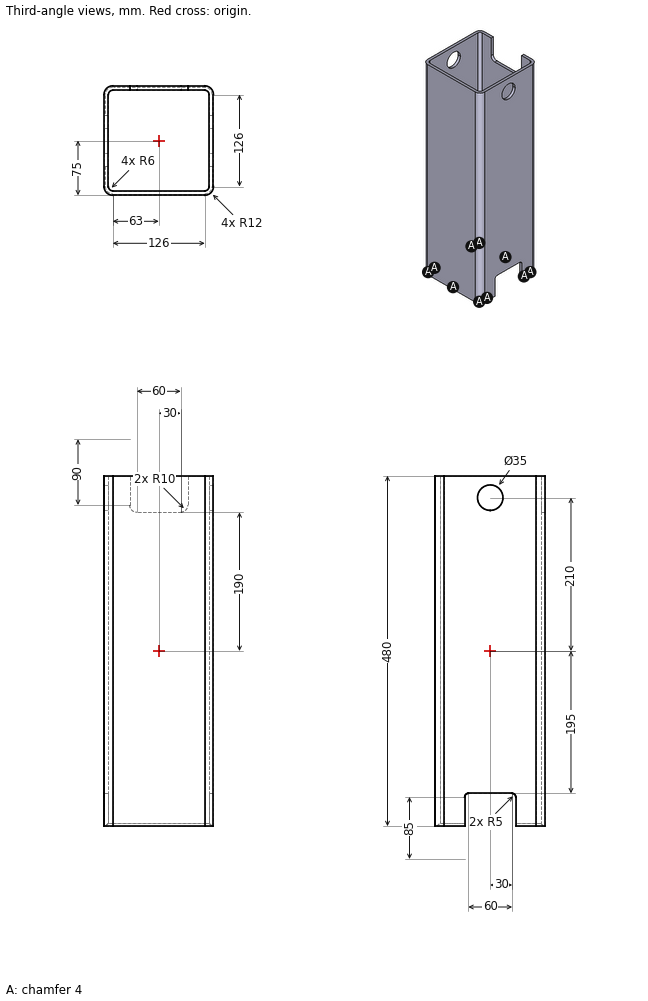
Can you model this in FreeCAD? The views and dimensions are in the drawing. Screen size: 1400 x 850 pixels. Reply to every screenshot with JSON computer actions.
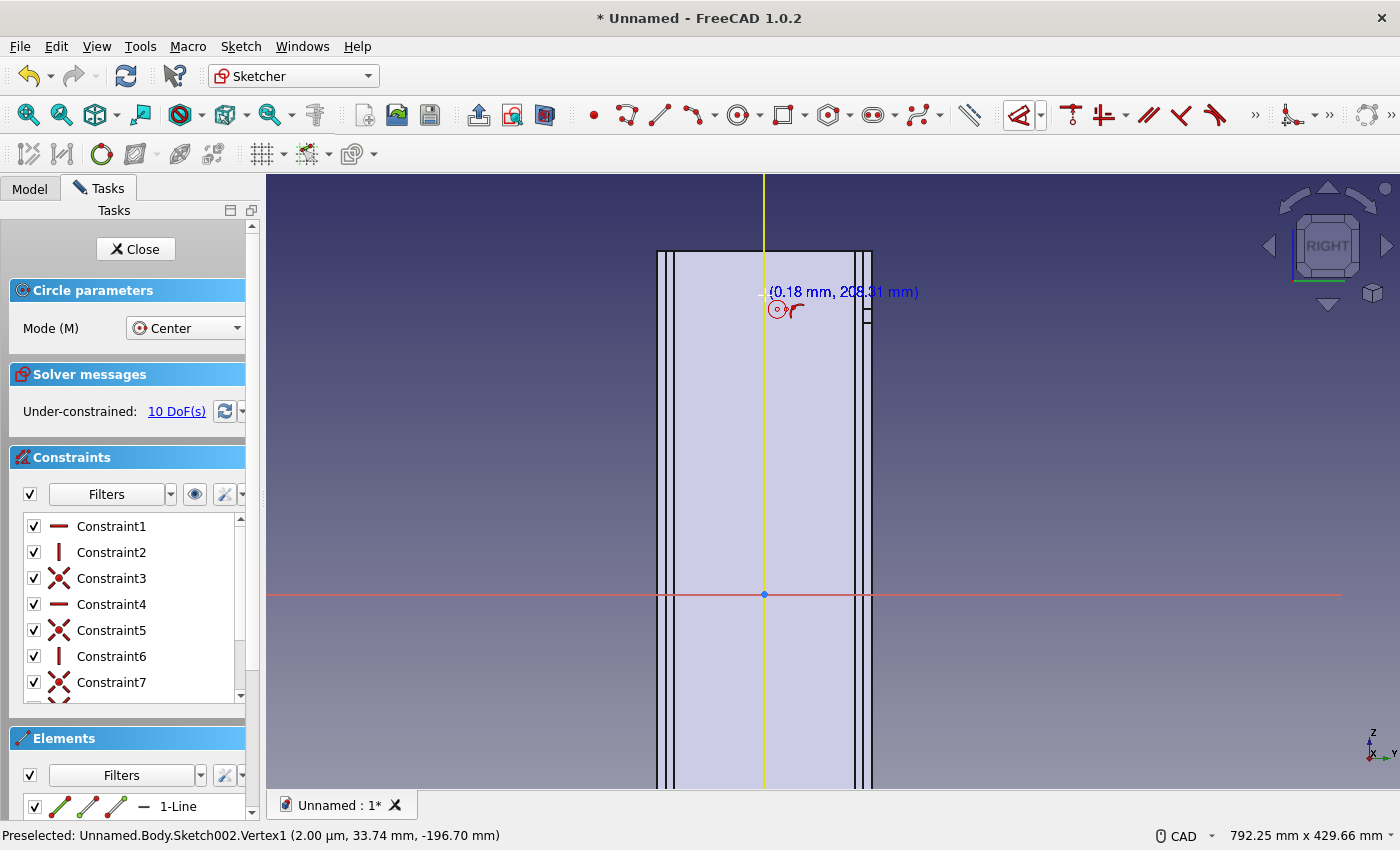
{"action": "left_click", "coordinate": [764, 294]}
{"action": "mouse_move", "coordinate": [782, 277]}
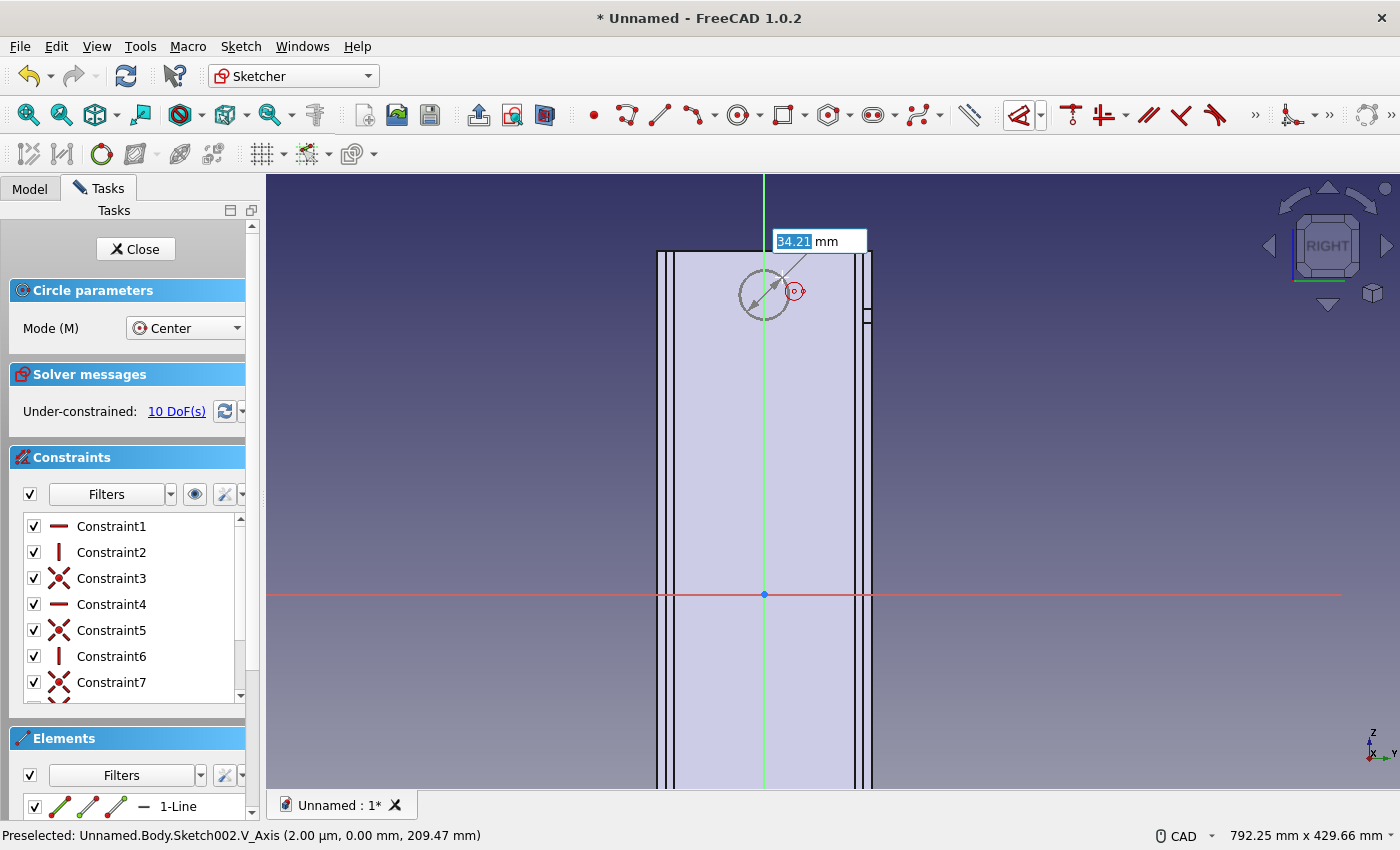
{"action": "type", "text": "35"}
{"action": "key", "text": "Return"}
{"action": "key", "text": "Escape"}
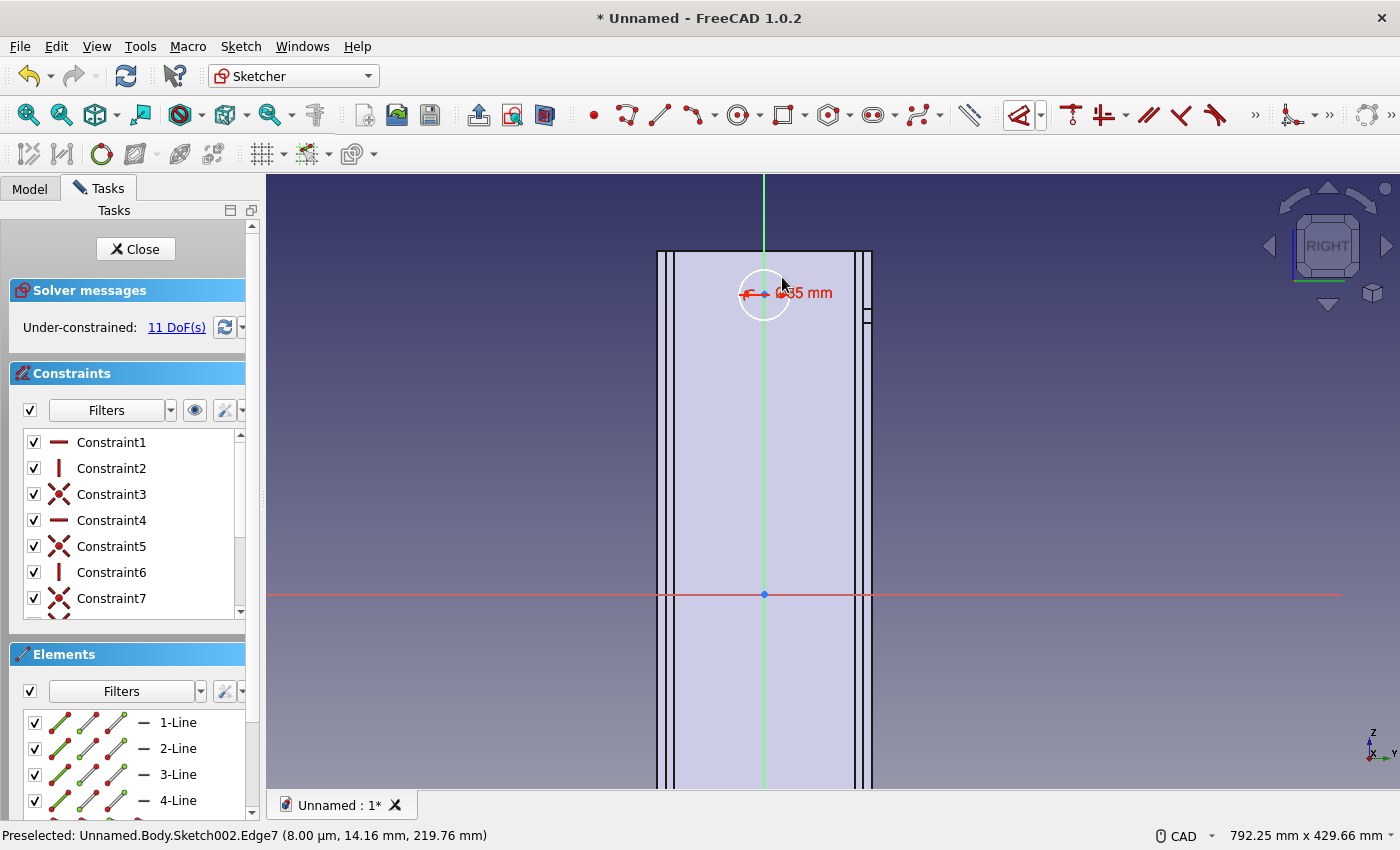
{"action": "scroll", "coordinate": [765, 294], "scroll_direction": "down", "scroll_amount": 3}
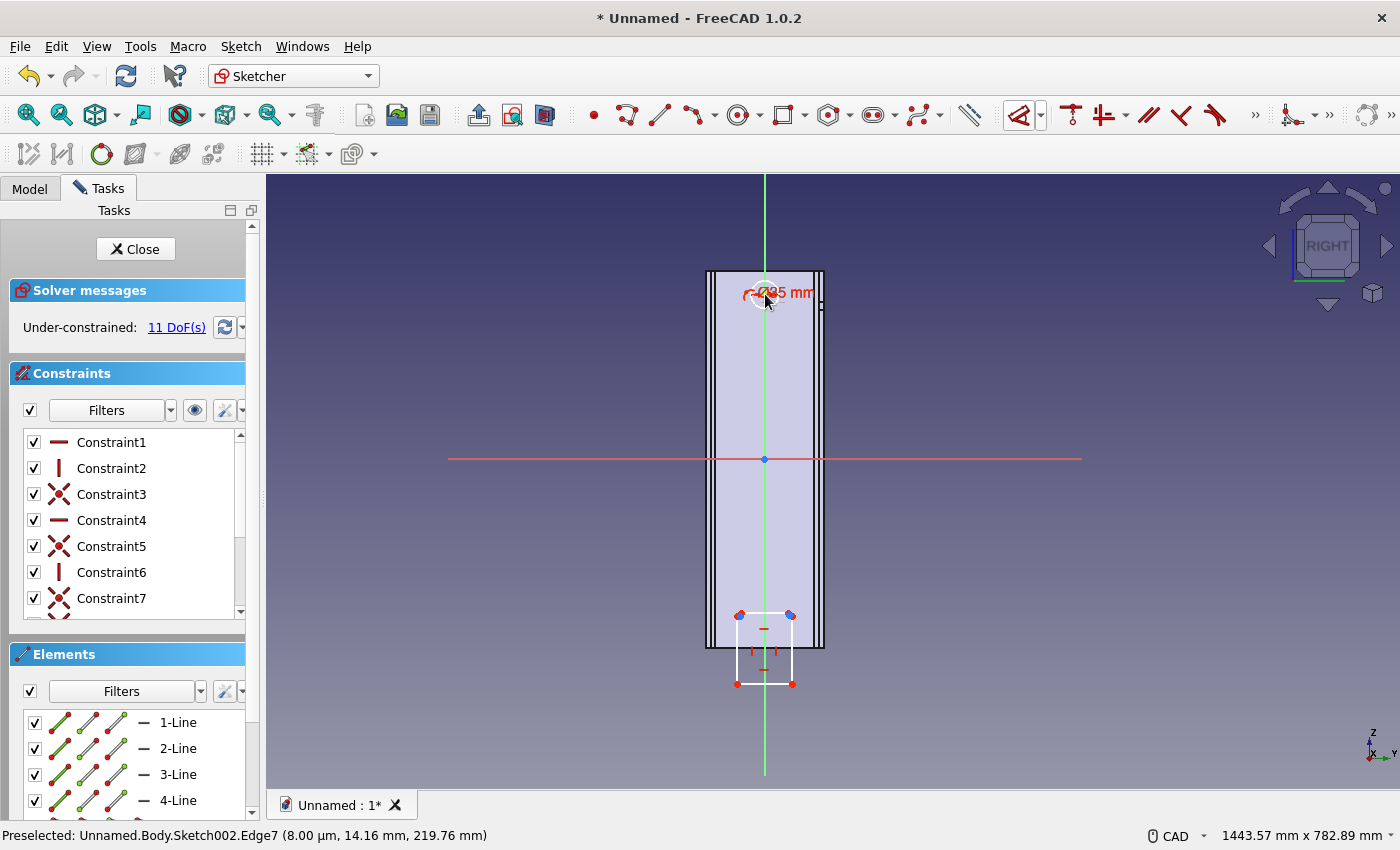
{"action": "scroll", "coordinate": [774, 613], "scroll_direction": "up", "scroll_amount": 2}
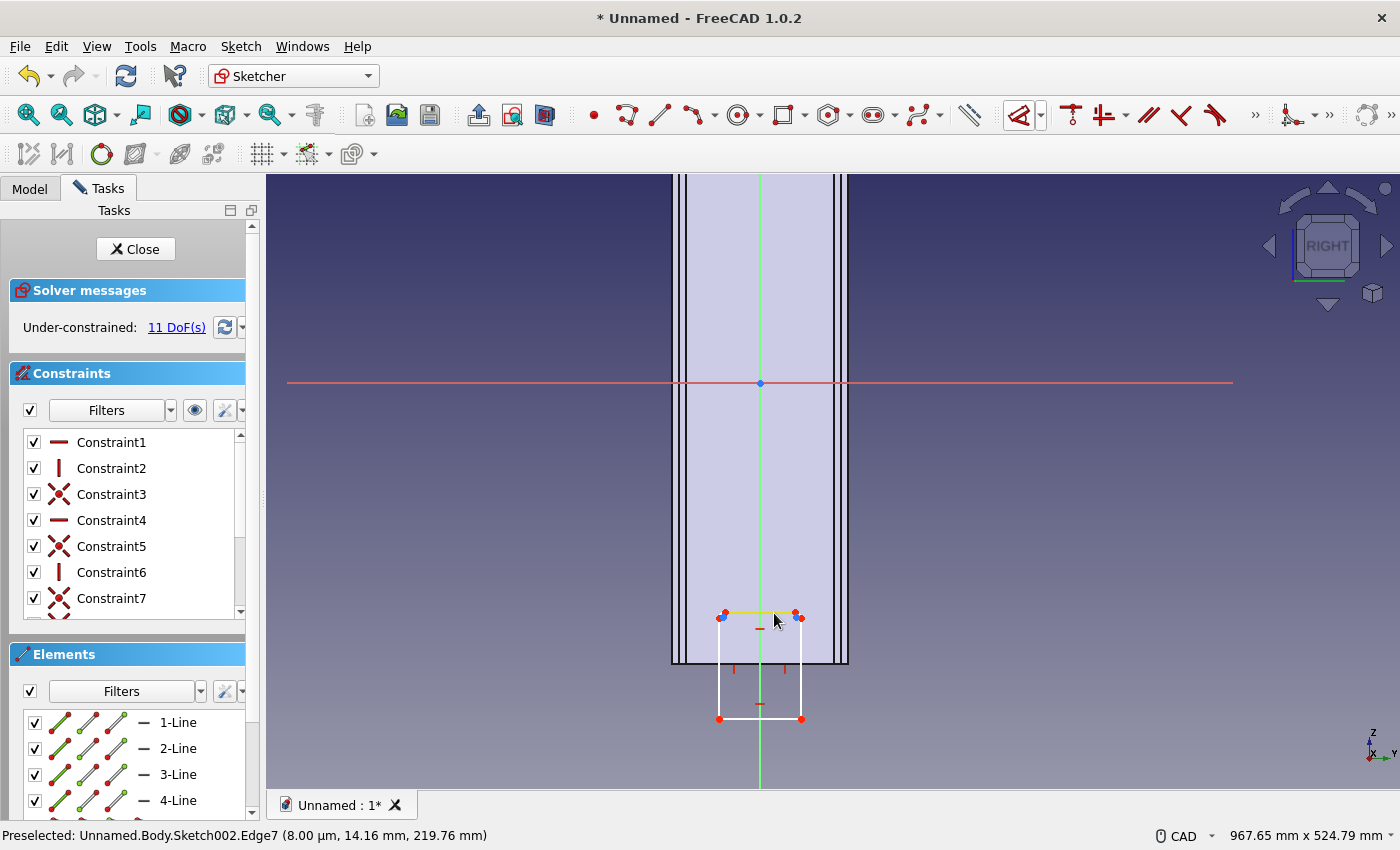
{"action": "left_click", "coordinate": [774, 613]}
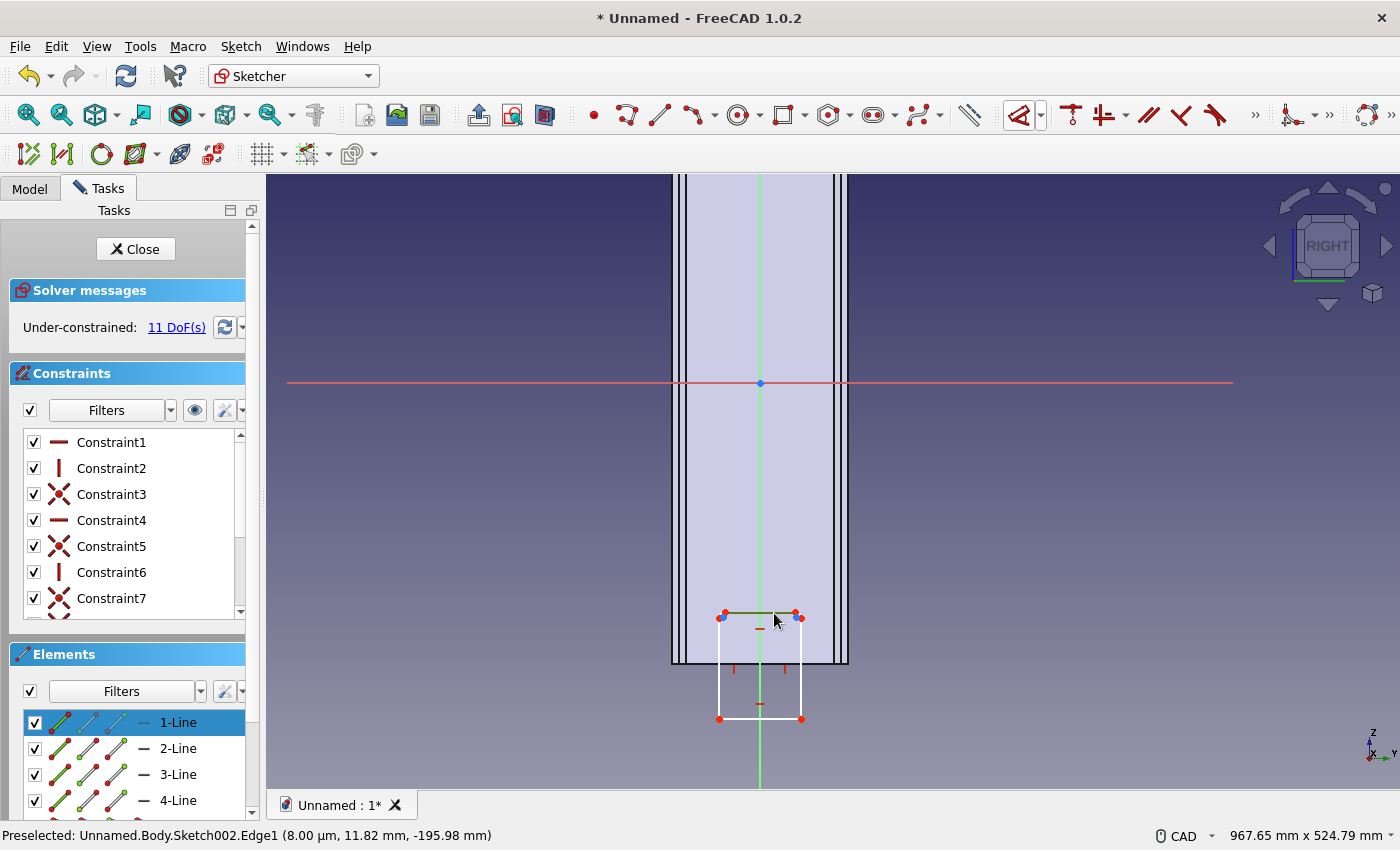
{"action": "scroll", "coordinate": [721, 614], "scroll_direction": "up", "scroll_amount": 6}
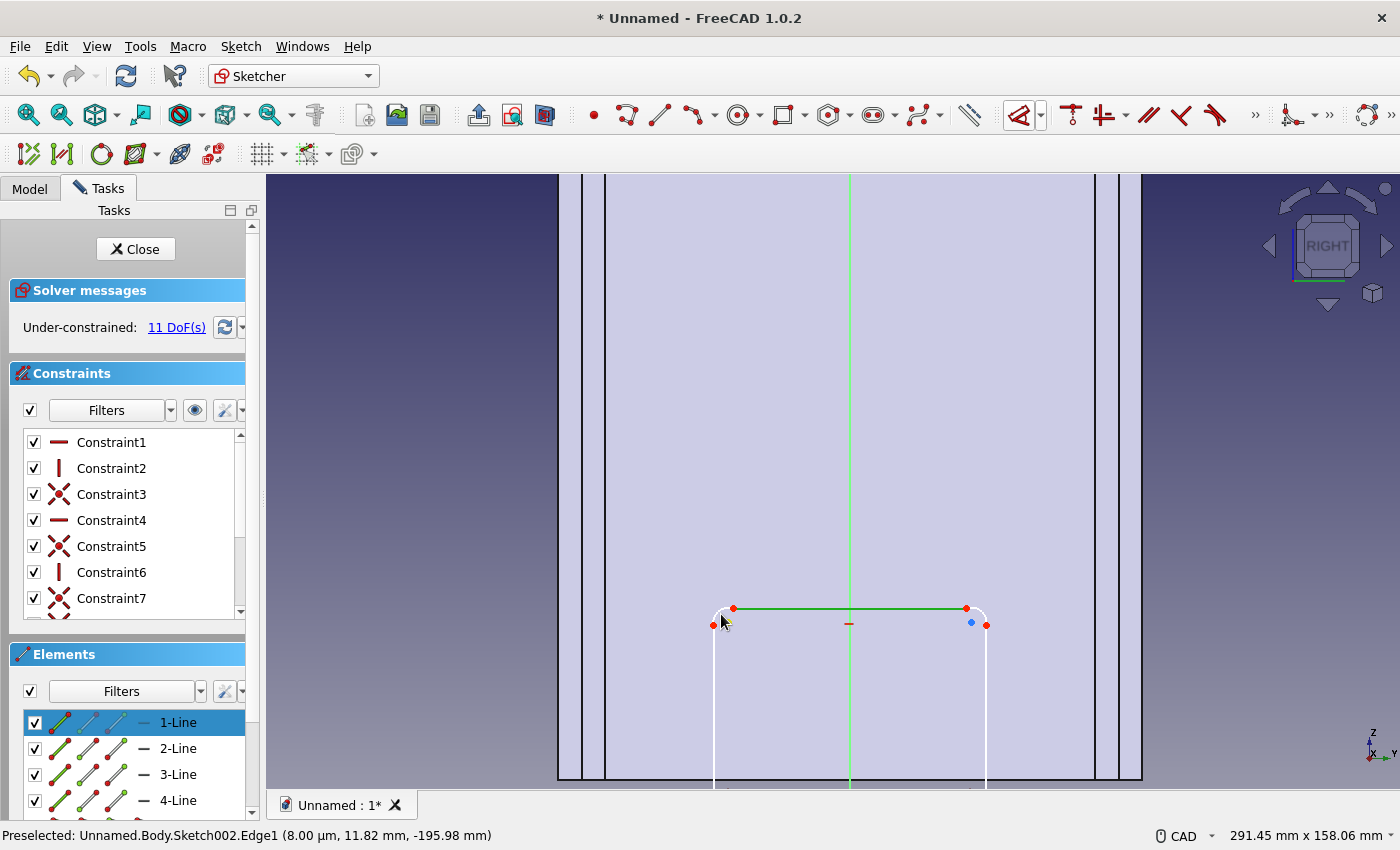
{"action": "left_click", "coordinate": [718, 611]}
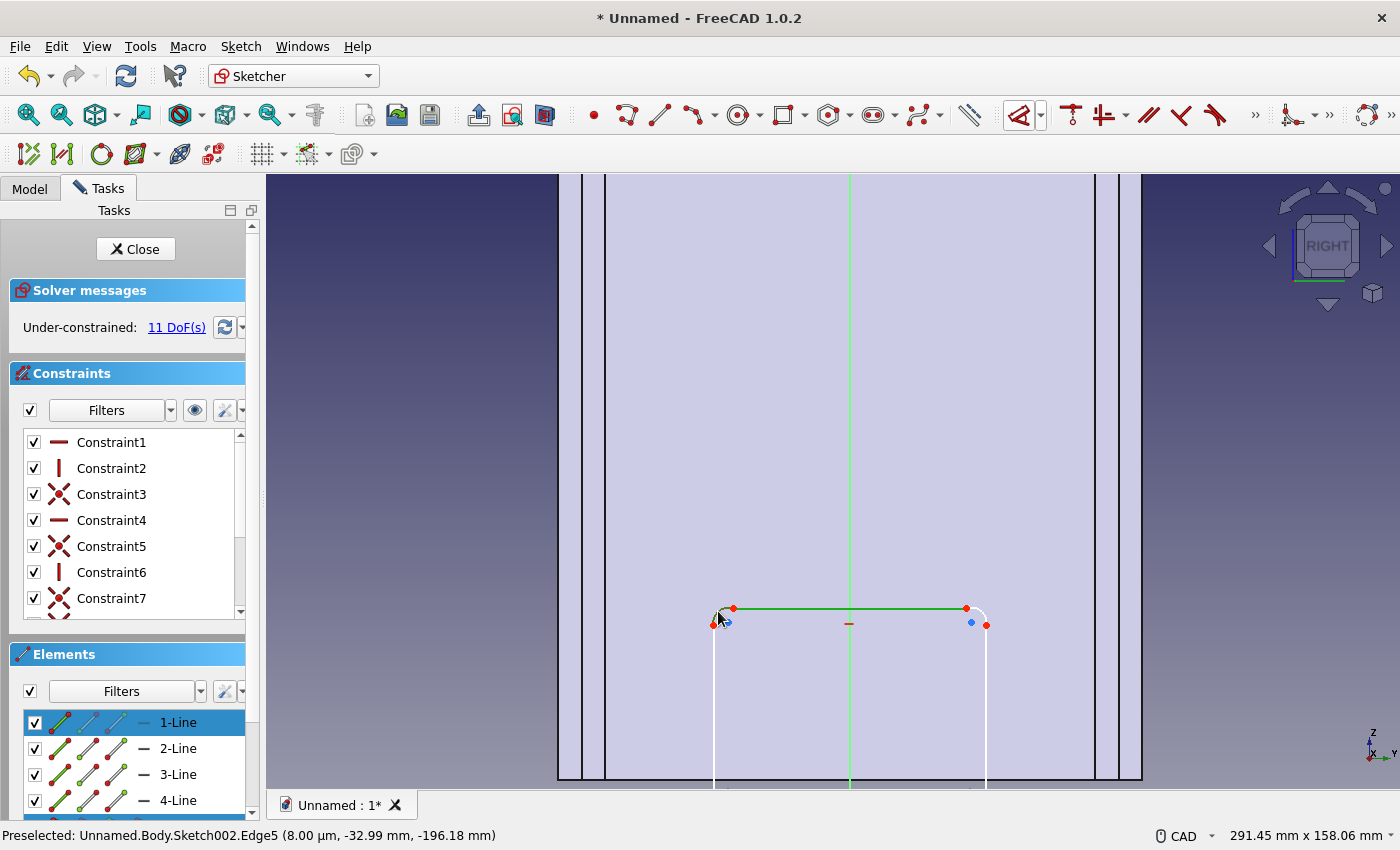
{"action": "key", "text": "t"}